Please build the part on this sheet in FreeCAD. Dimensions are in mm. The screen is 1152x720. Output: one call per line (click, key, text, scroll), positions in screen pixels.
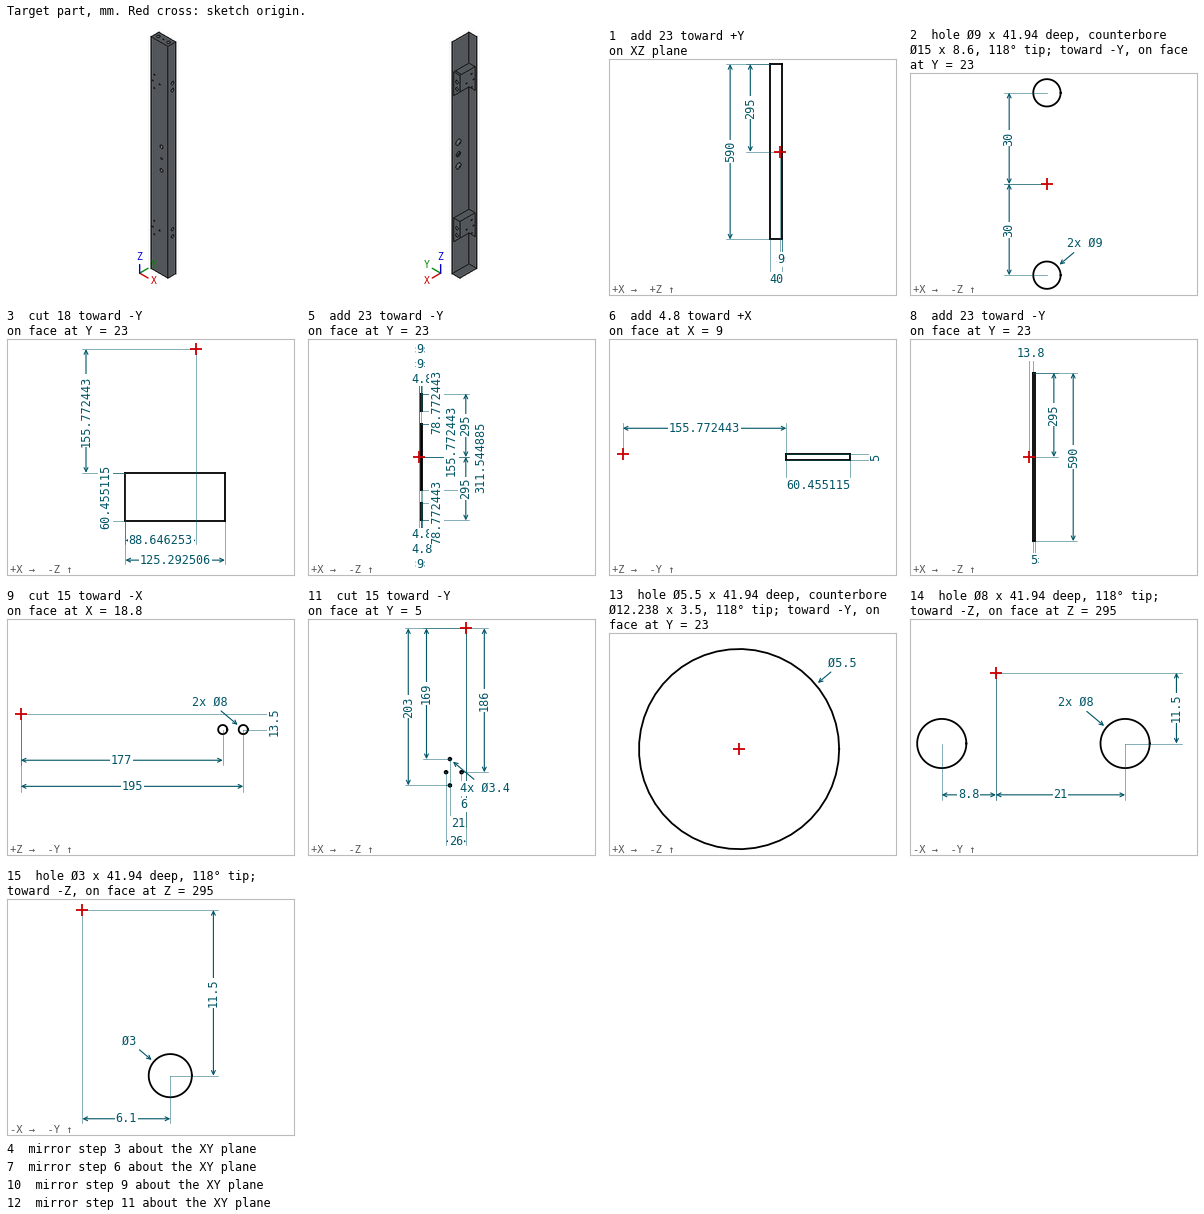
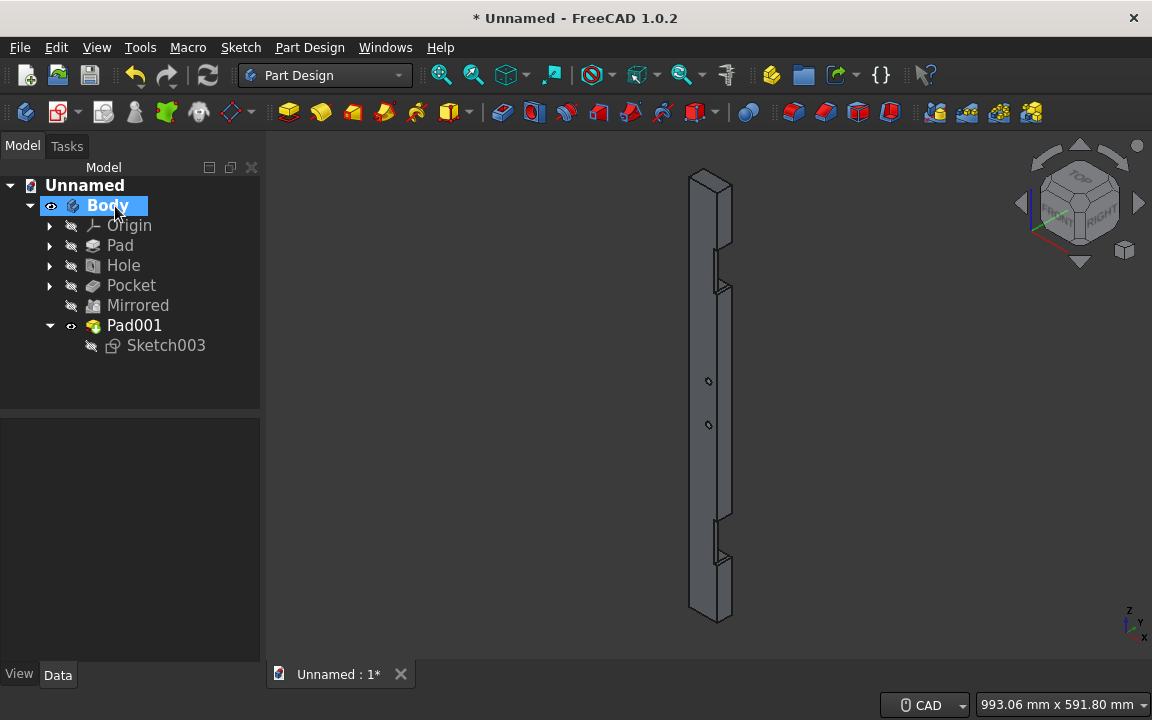
scroll(716, 263, up, 9)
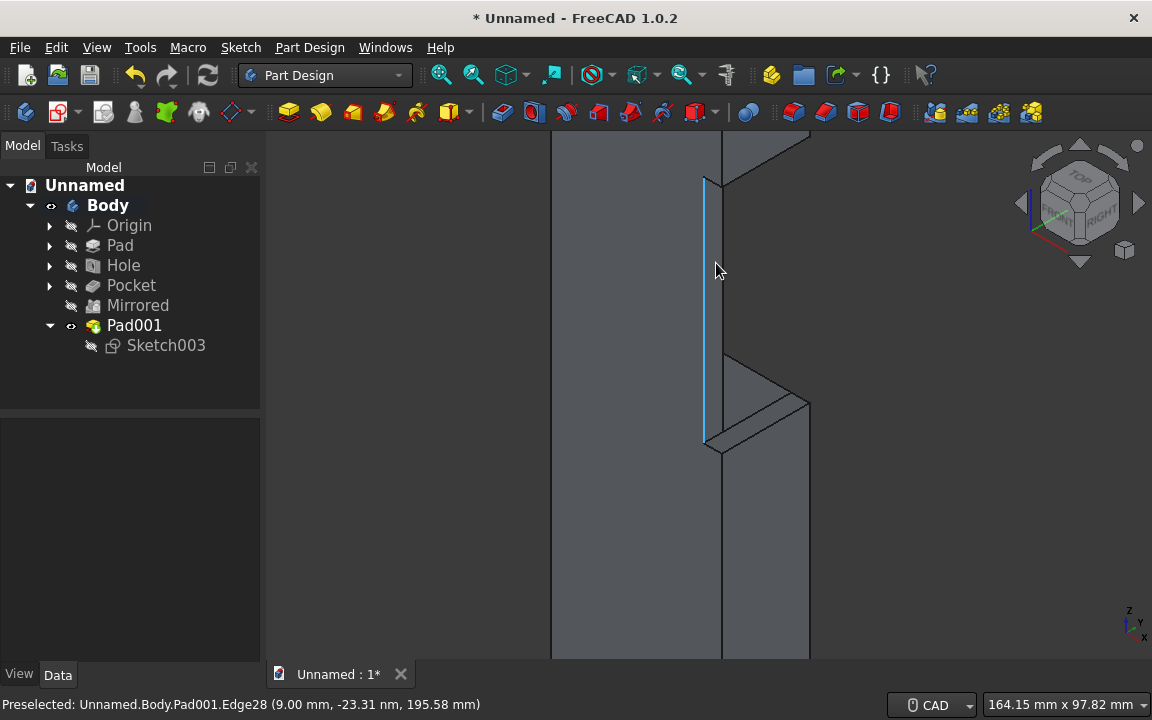
click(713, 265)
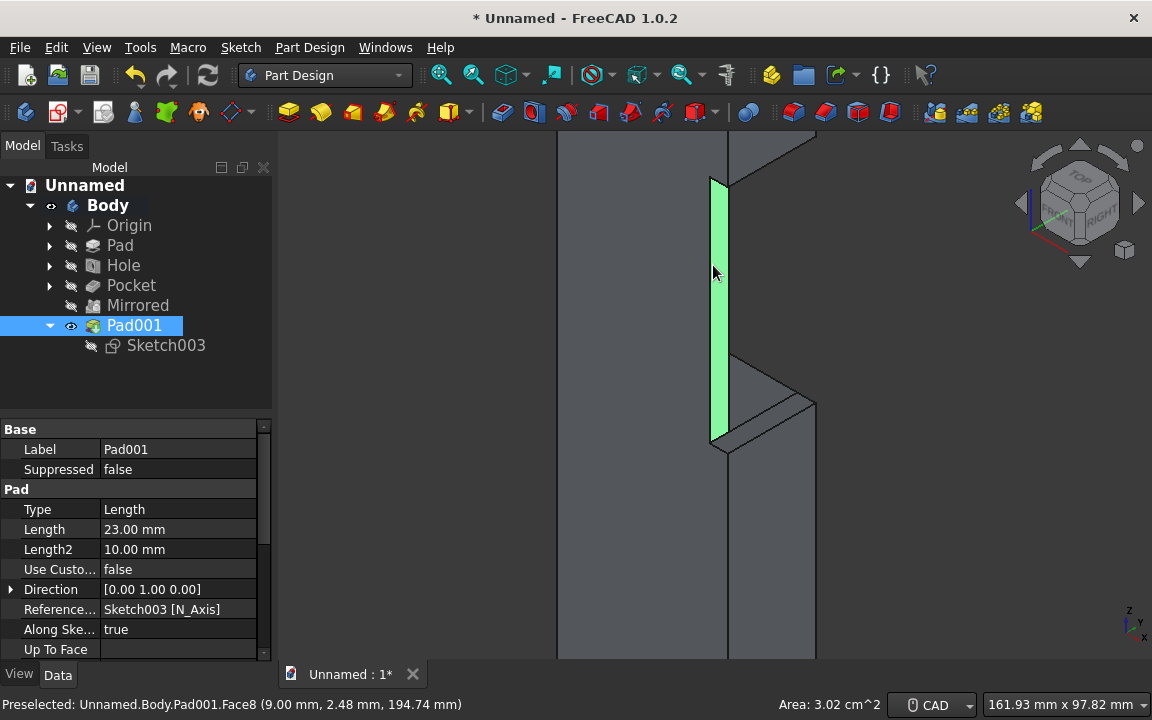
click(58, 112)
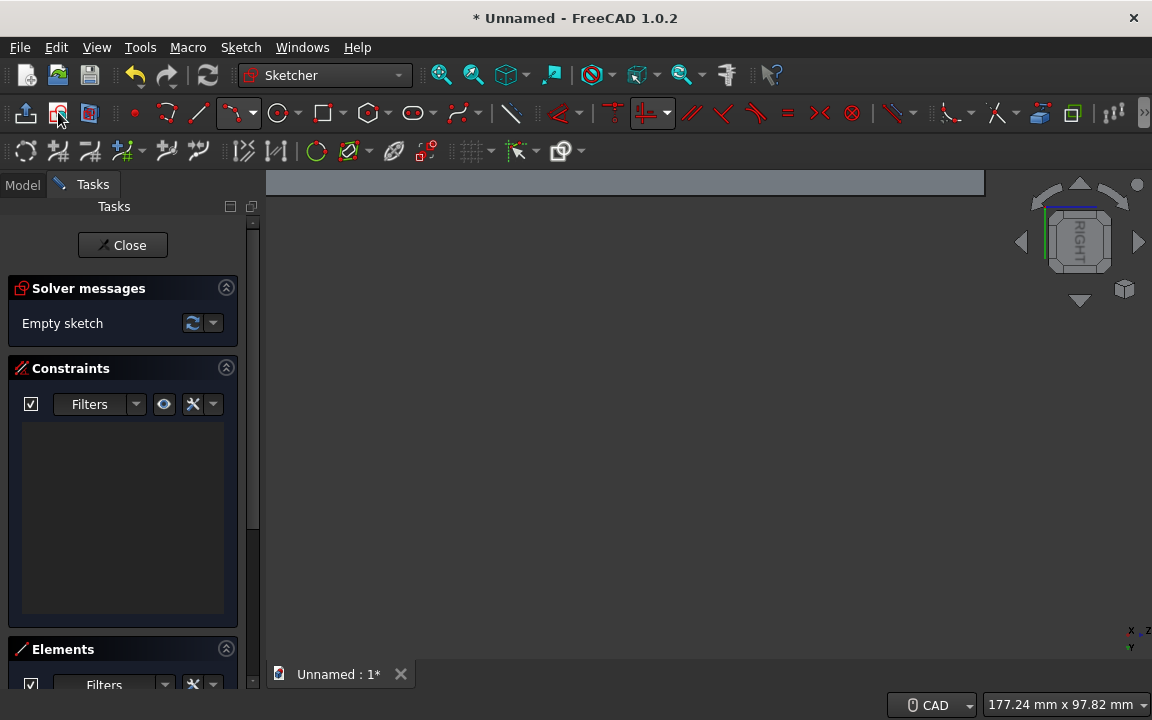
scroll(640, 414, down, 5)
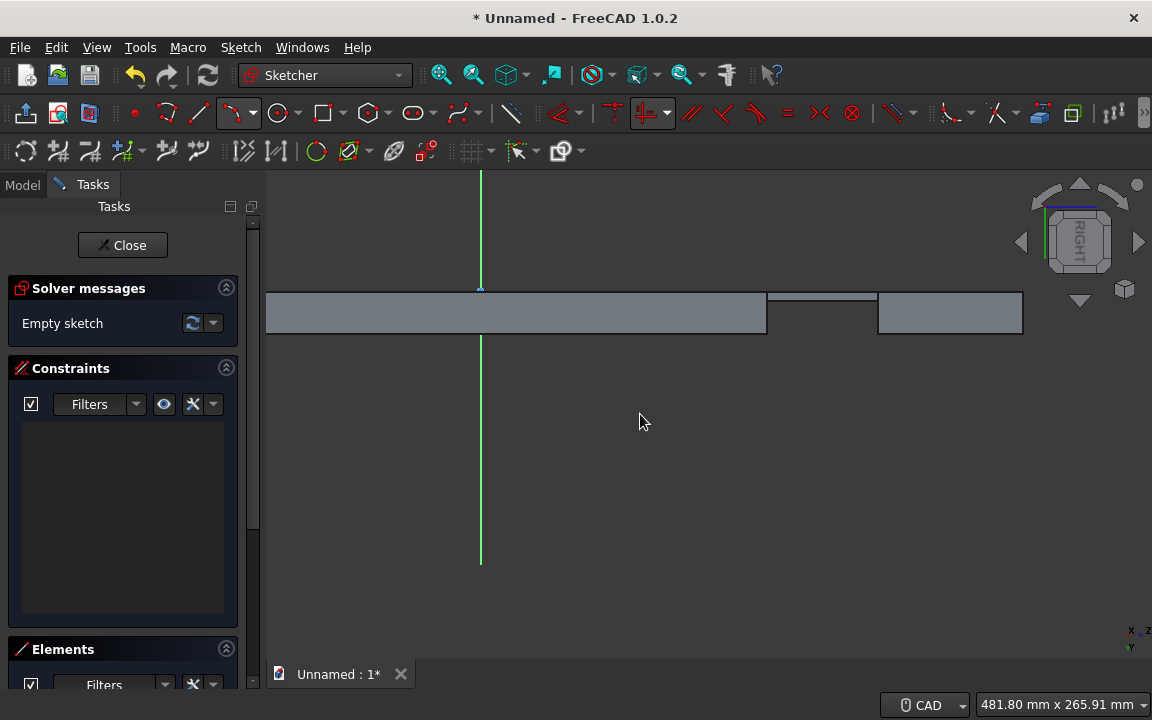
scroll(882, 258, up, 7)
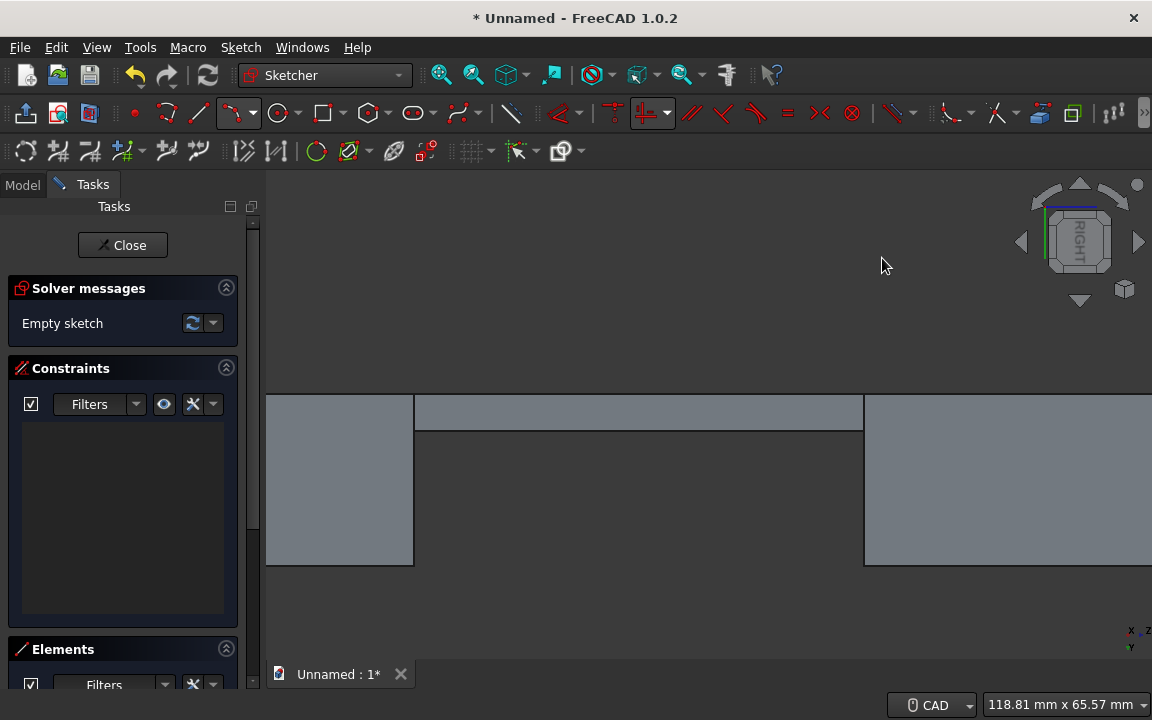
click(324, 114)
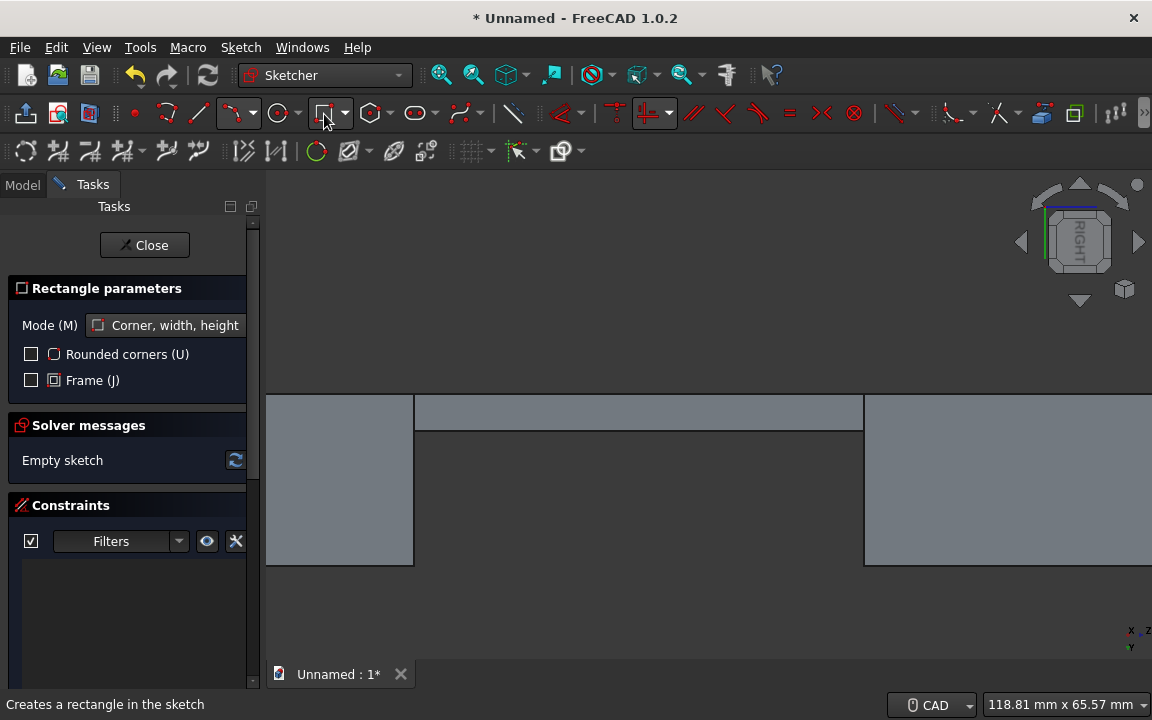
click(414, 394)
click(864, 431)
key(Escape)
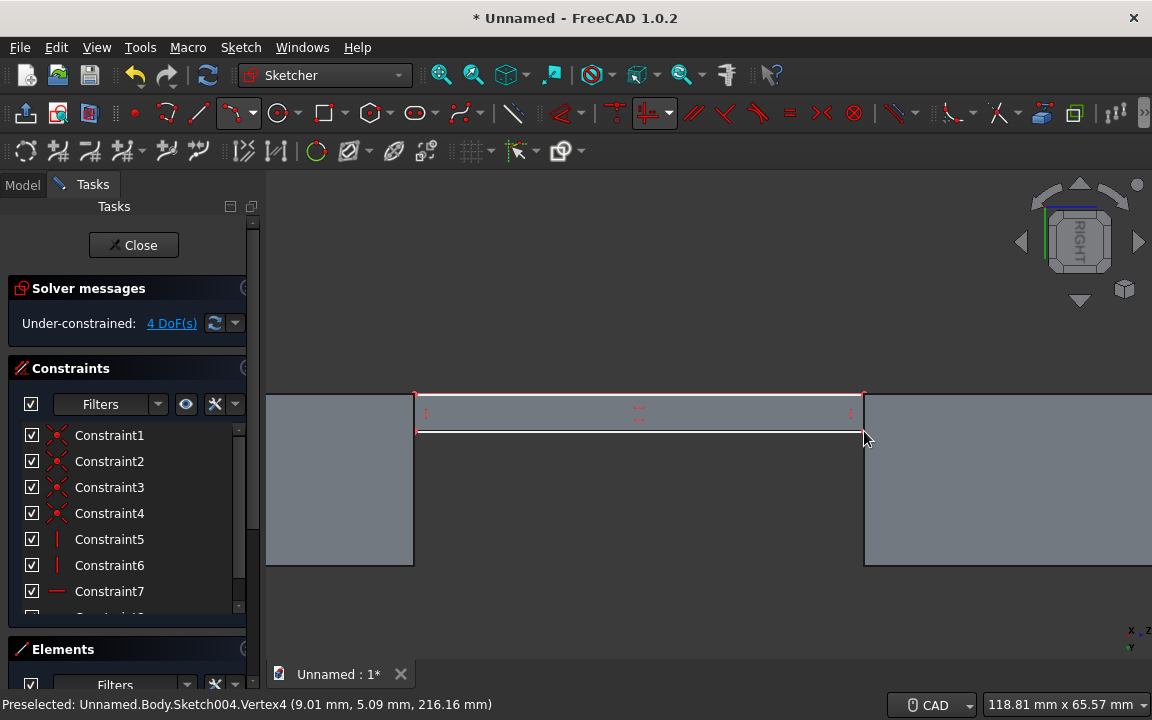
click(414, 395)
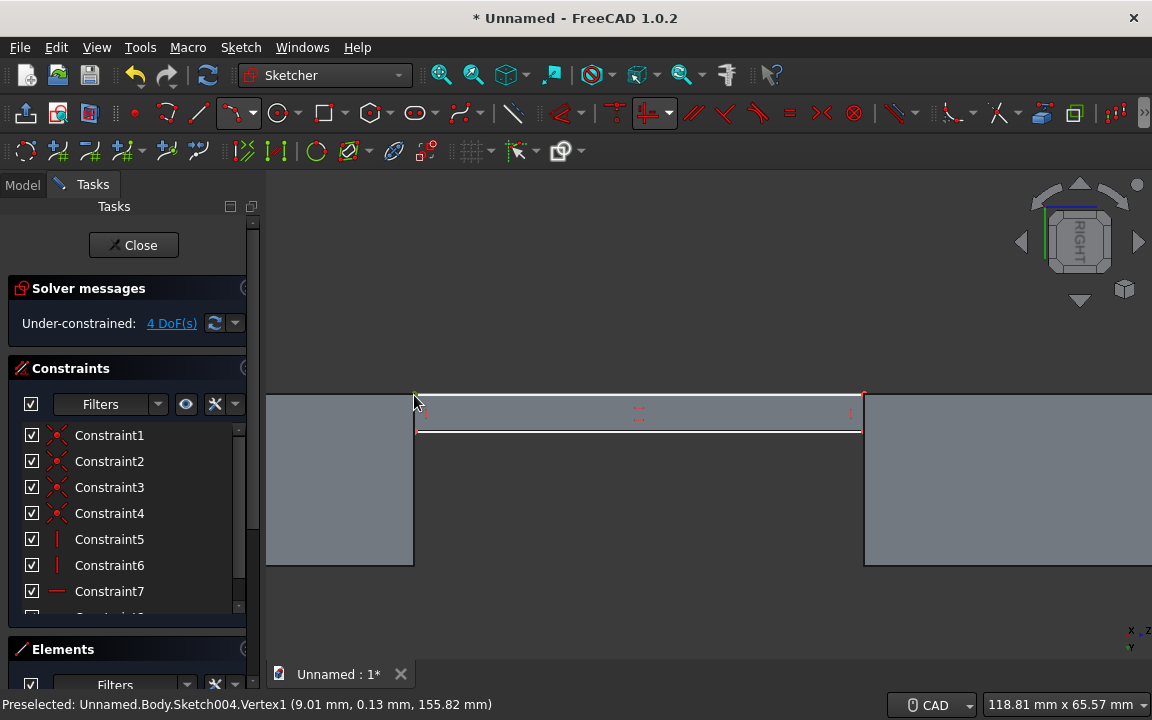
click(344, 394)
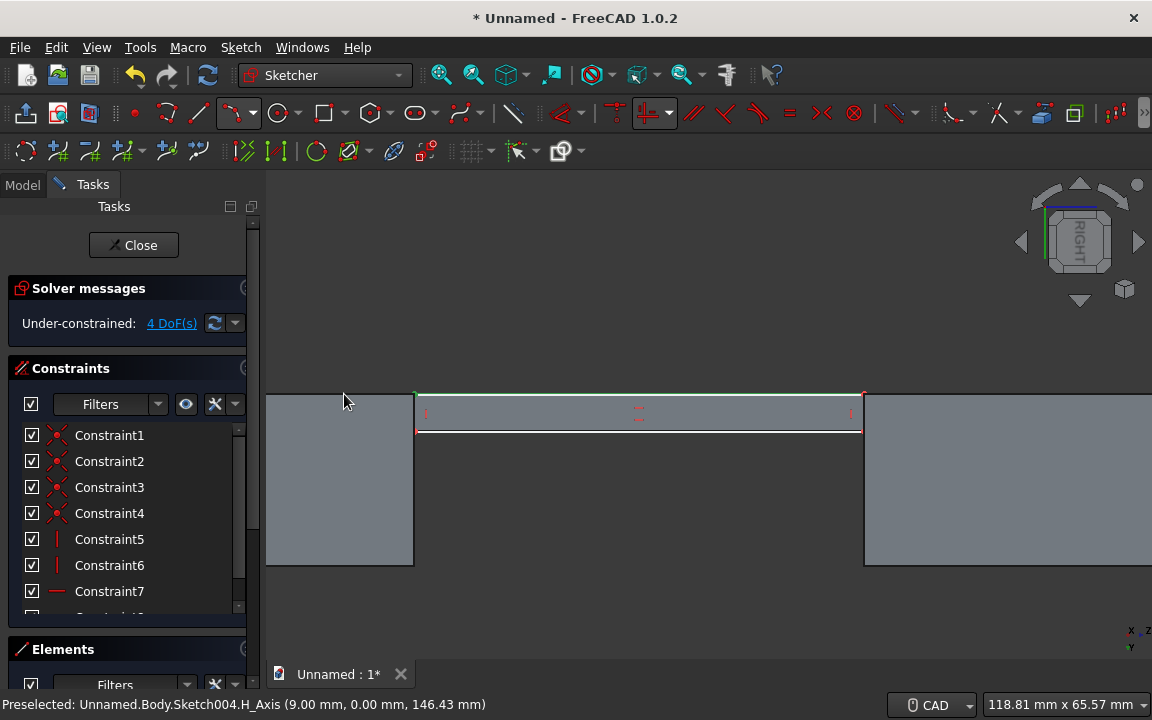
click(616, 114)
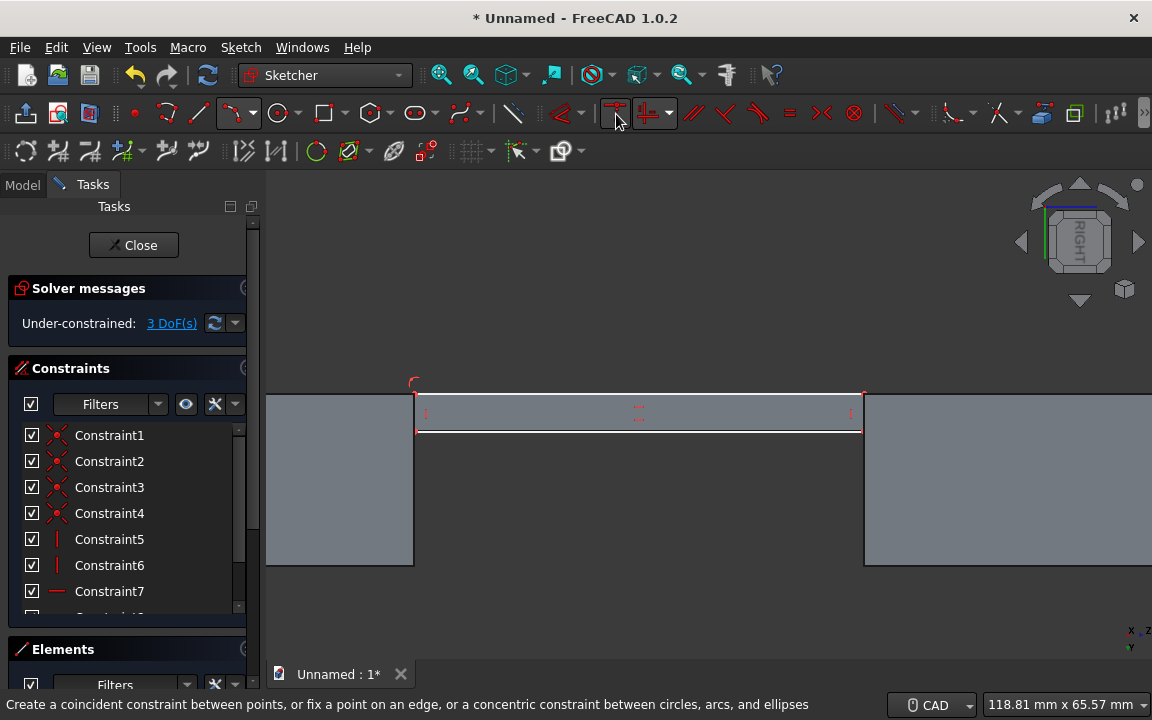
click(560, 114)